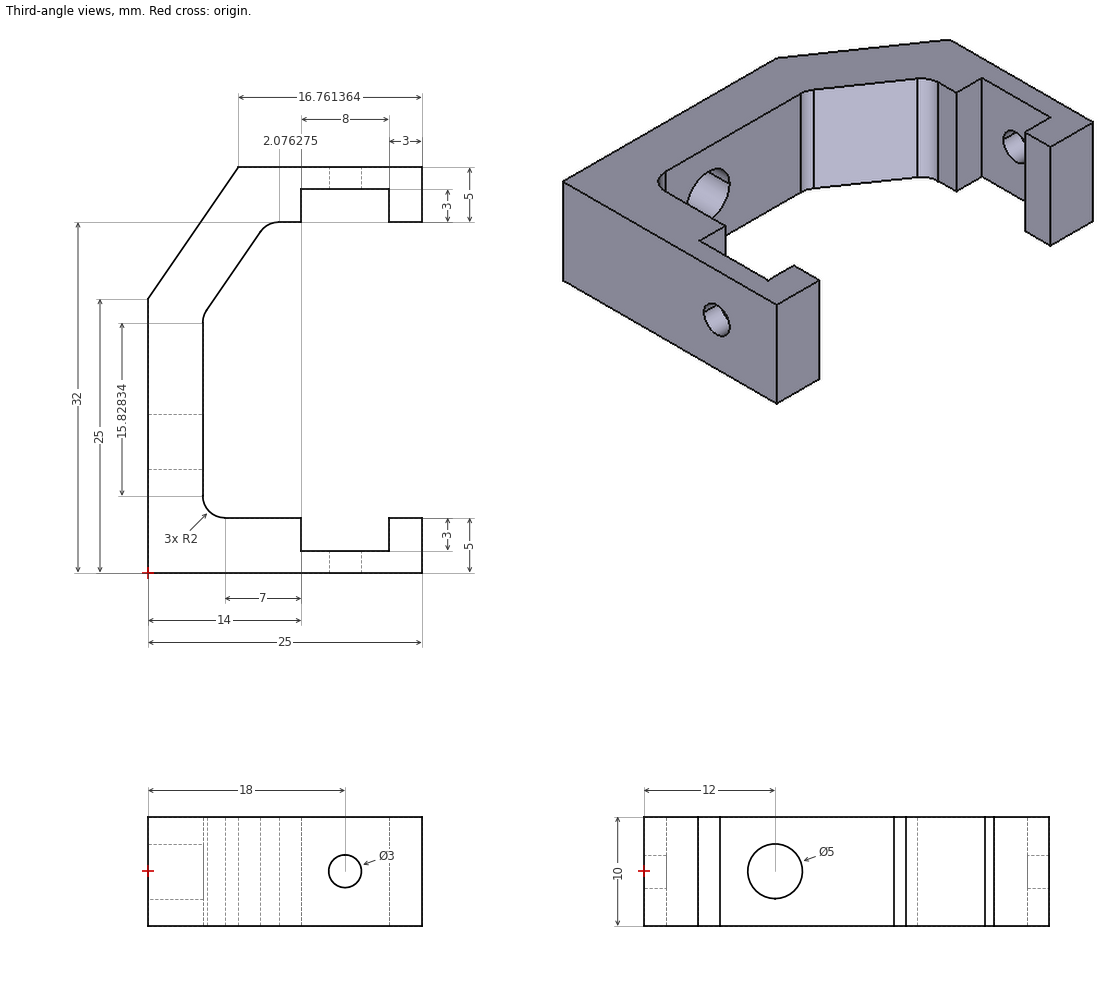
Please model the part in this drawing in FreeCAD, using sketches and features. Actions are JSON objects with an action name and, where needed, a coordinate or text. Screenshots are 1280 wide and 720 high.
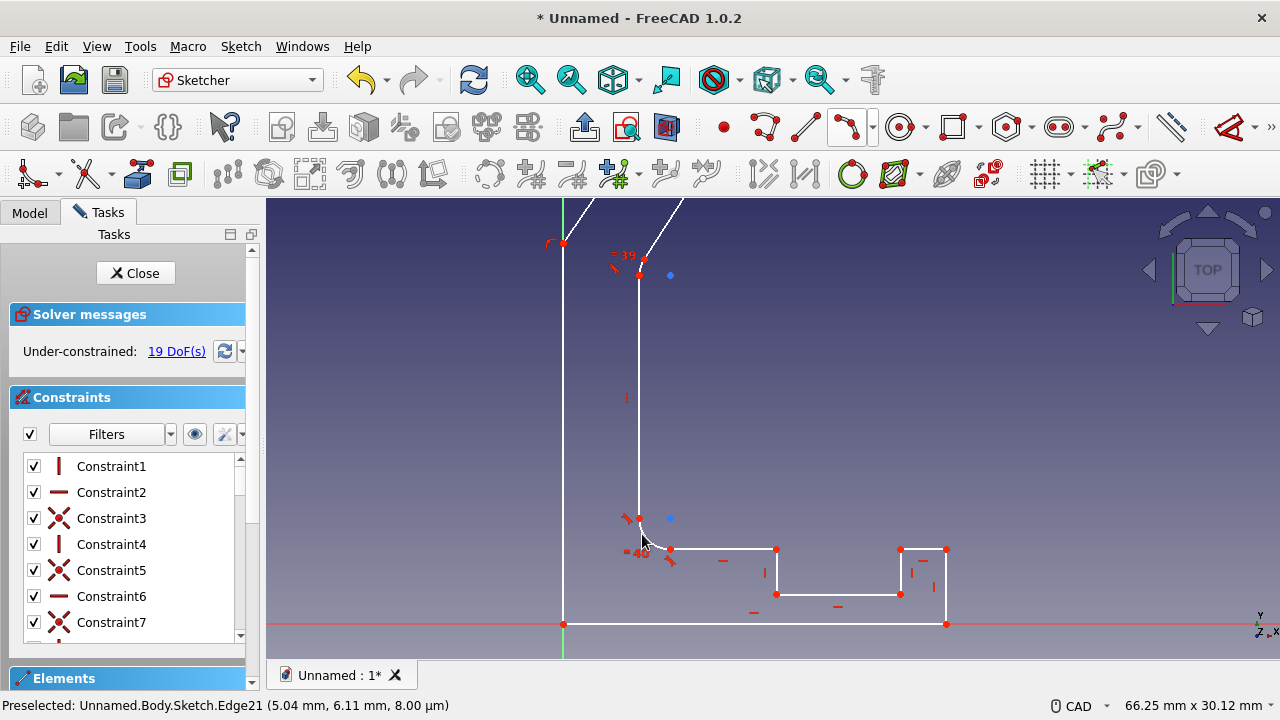
{"action": "left_click", "coordinate": [1228, 128]}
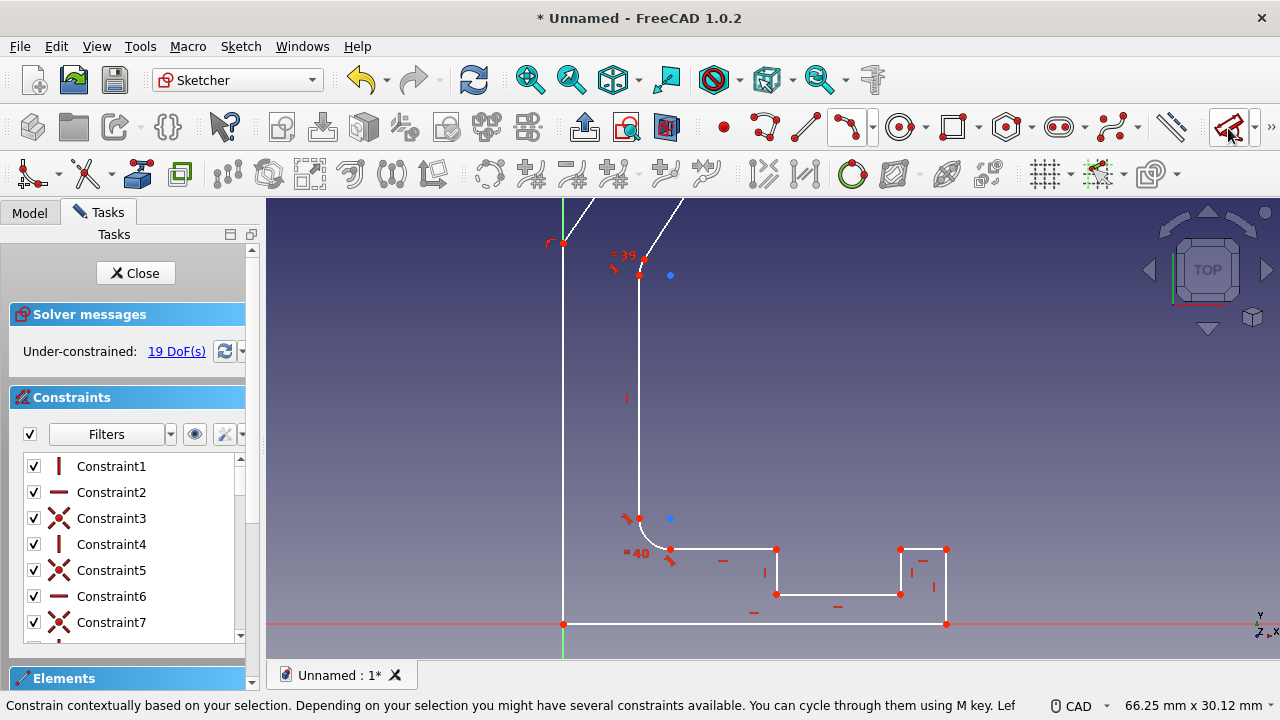
{"action": "scroll", "coordinate": [641, 267], "scroll_direction": "up", "scroll_amount": 3}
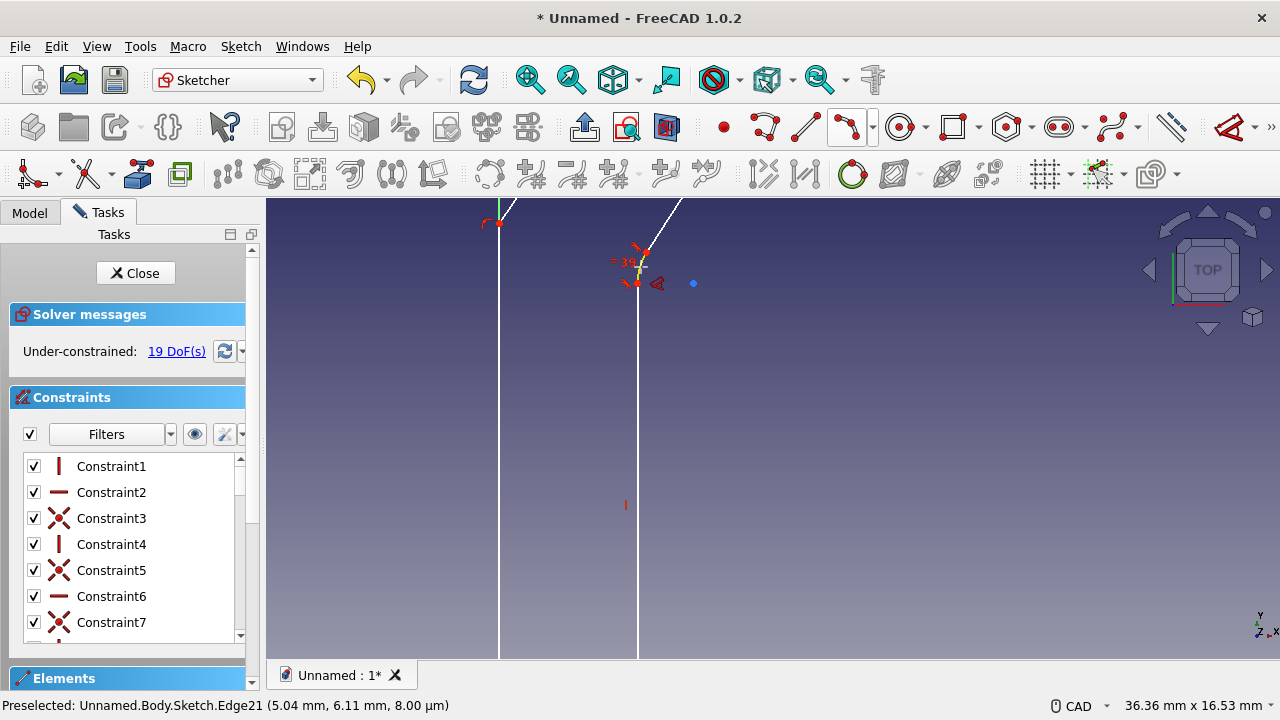
{"action": "left_click", "coordinate": [640, 267]}
{"action": "left_click", "coordinate": [609, 258]}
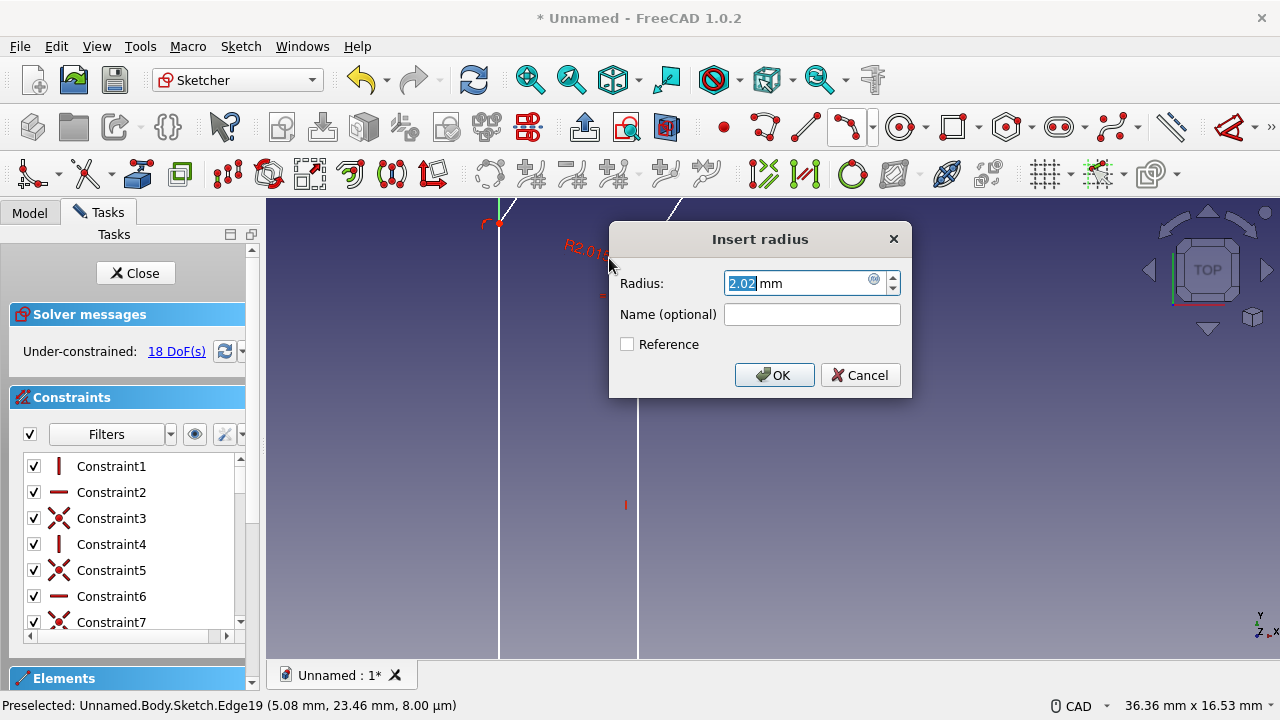
{"action": "type", "text": "2"}
{"action": "key", "text": "Return"}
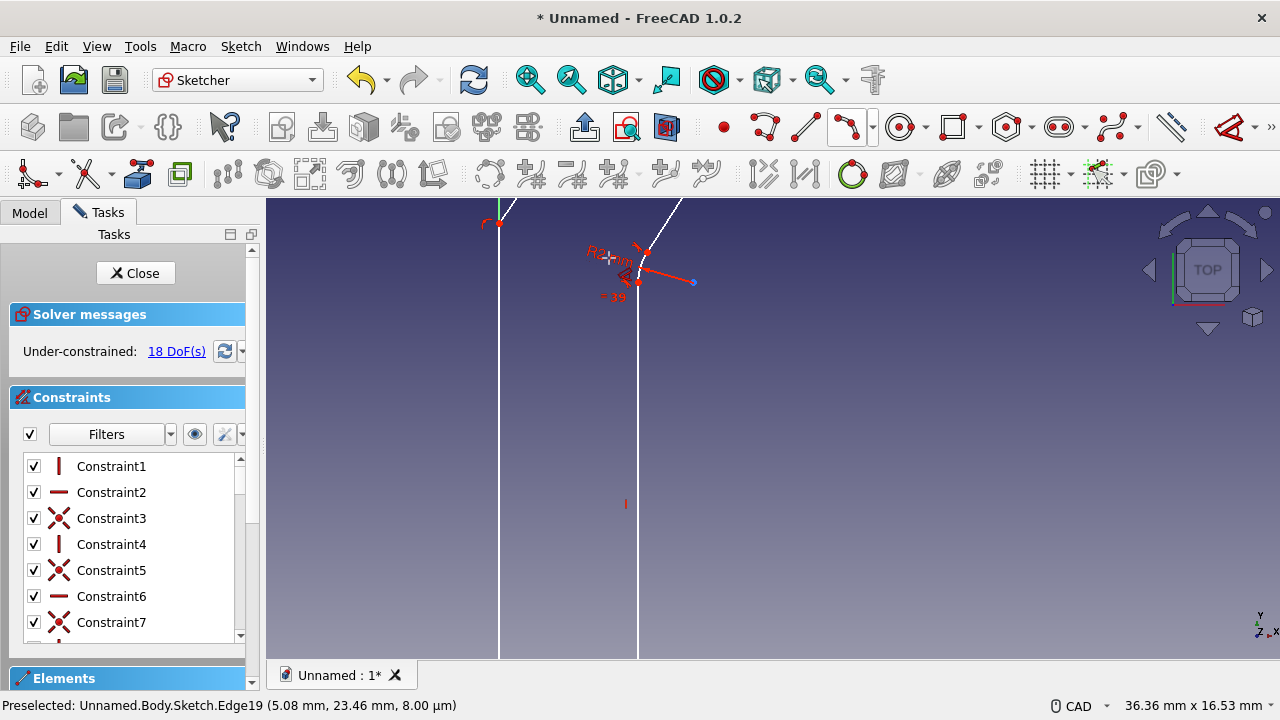
{"action": "scroll", "coordinate": [643, 440], "scroll_direction": "down", "scroll_amount": 6}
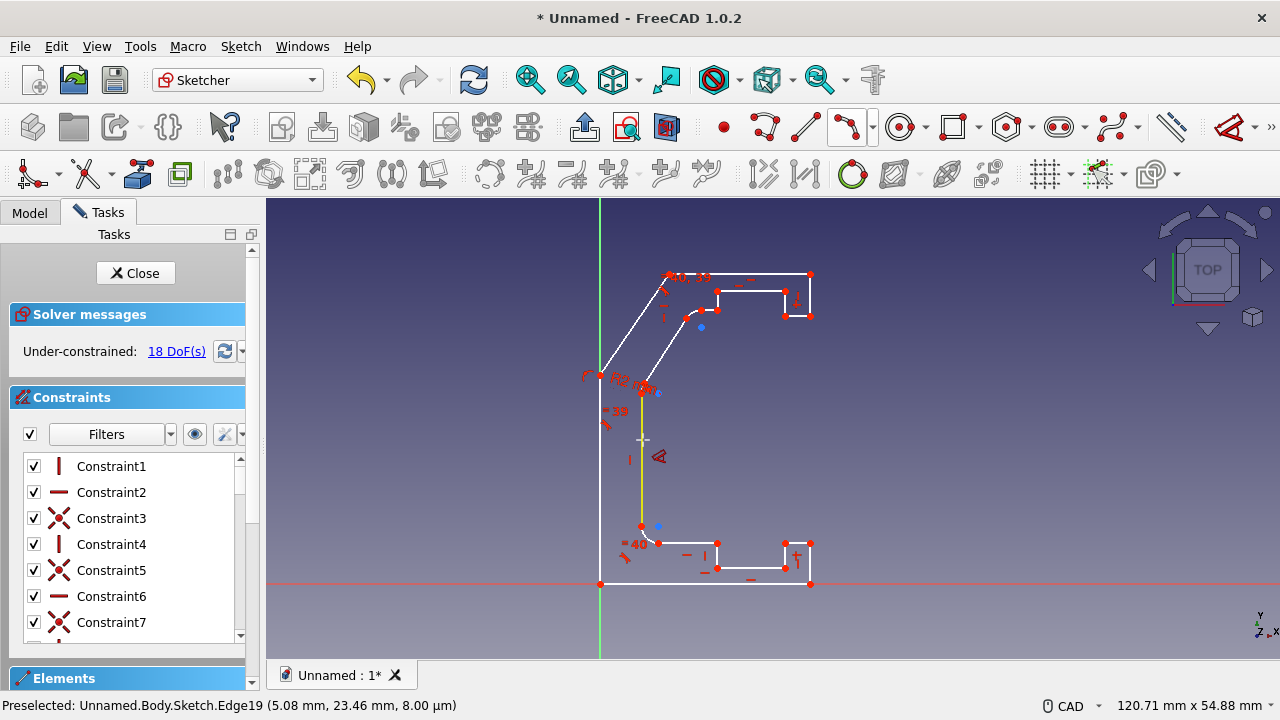
{"action": "scroll", "coordinate": [718, 305], "scroll_direction": "up", "scroll_amount": 5}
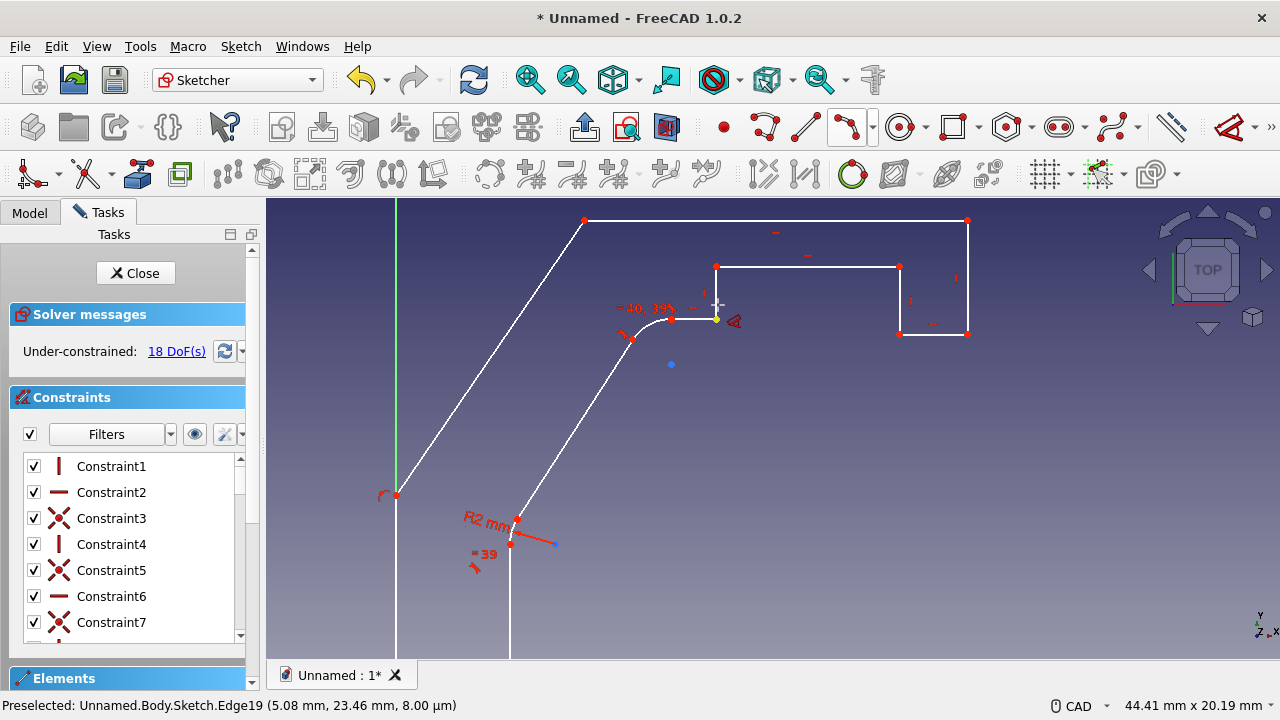
{"action": "left_click", "coordinate": [716, 303]}
{"action": "left_click", "coordinate": [750, 293]}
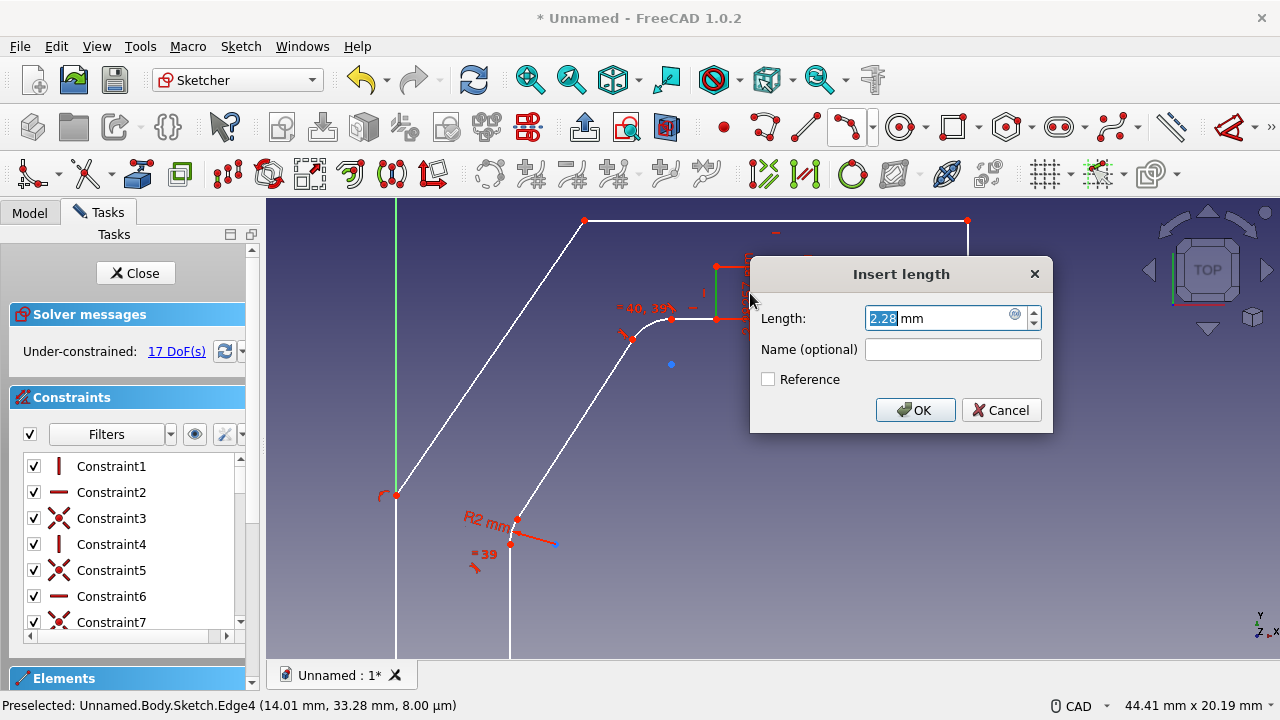
{"action": "type", "text": "3"}
{"action": "key", "text": "Return"}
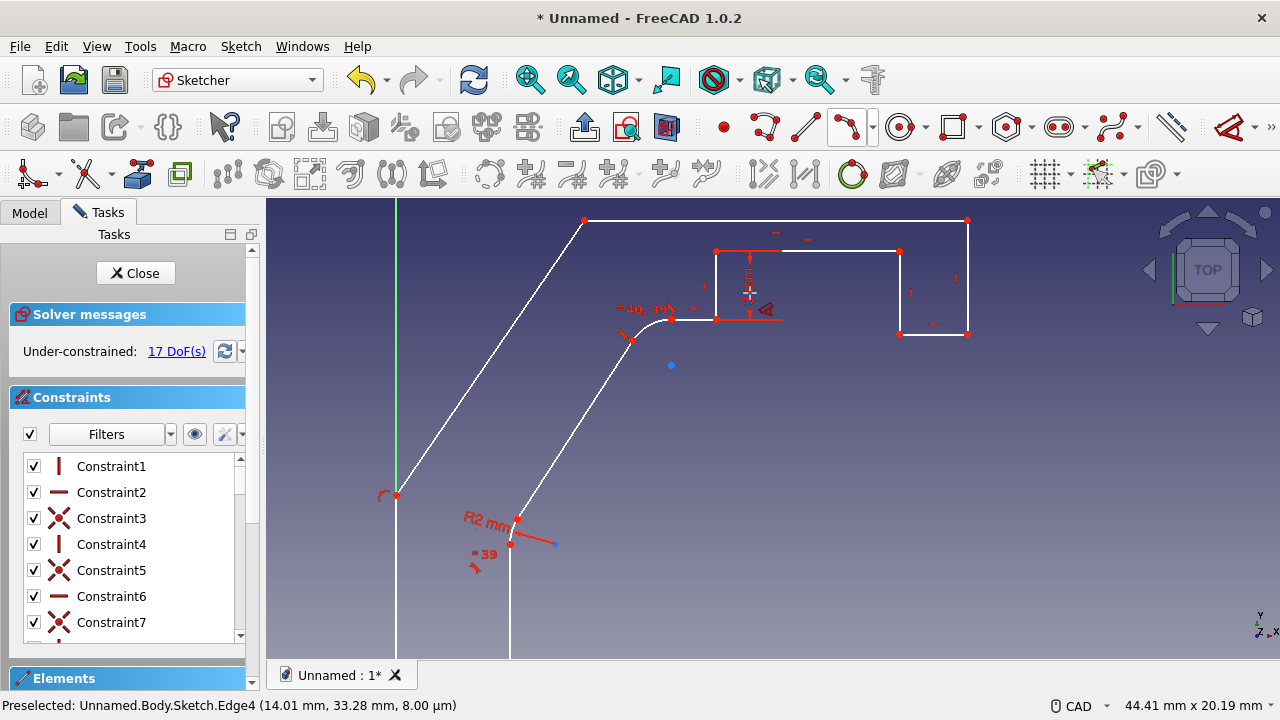
{"action": "left_click", "coordinate": [771, 251]}
{"action": "left_click", "coordinate": [850, 285]}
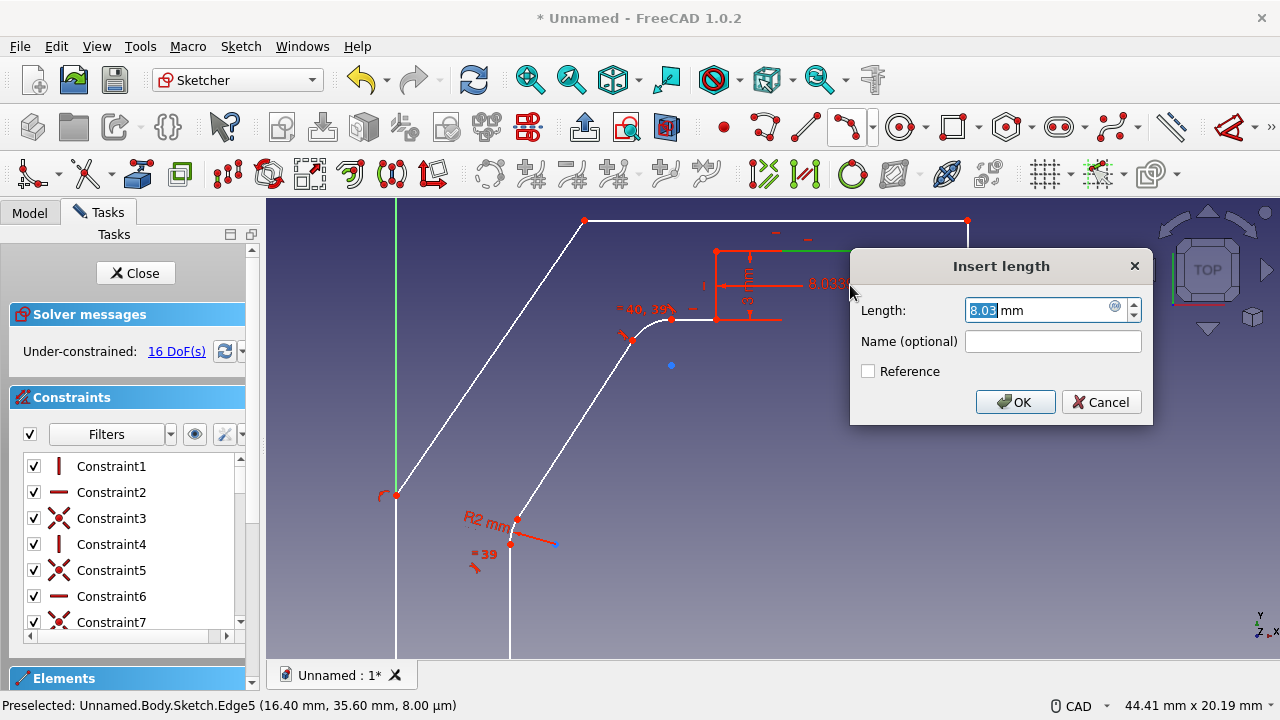
{"action": "type", "text": "8"}
{"action": "key", "text": "Return"}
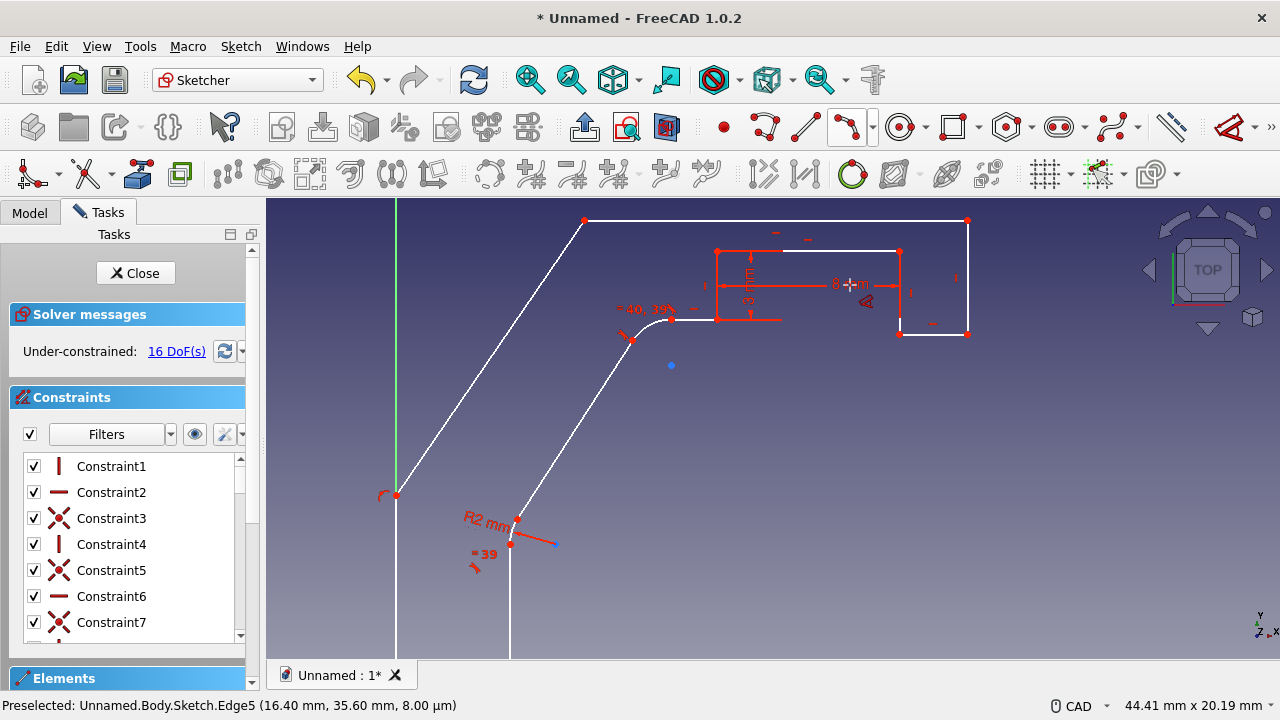
{"action": "left_click", "coordinate": [900, 276]}
{"action": "left_click", "coordinate": [934, 293]}